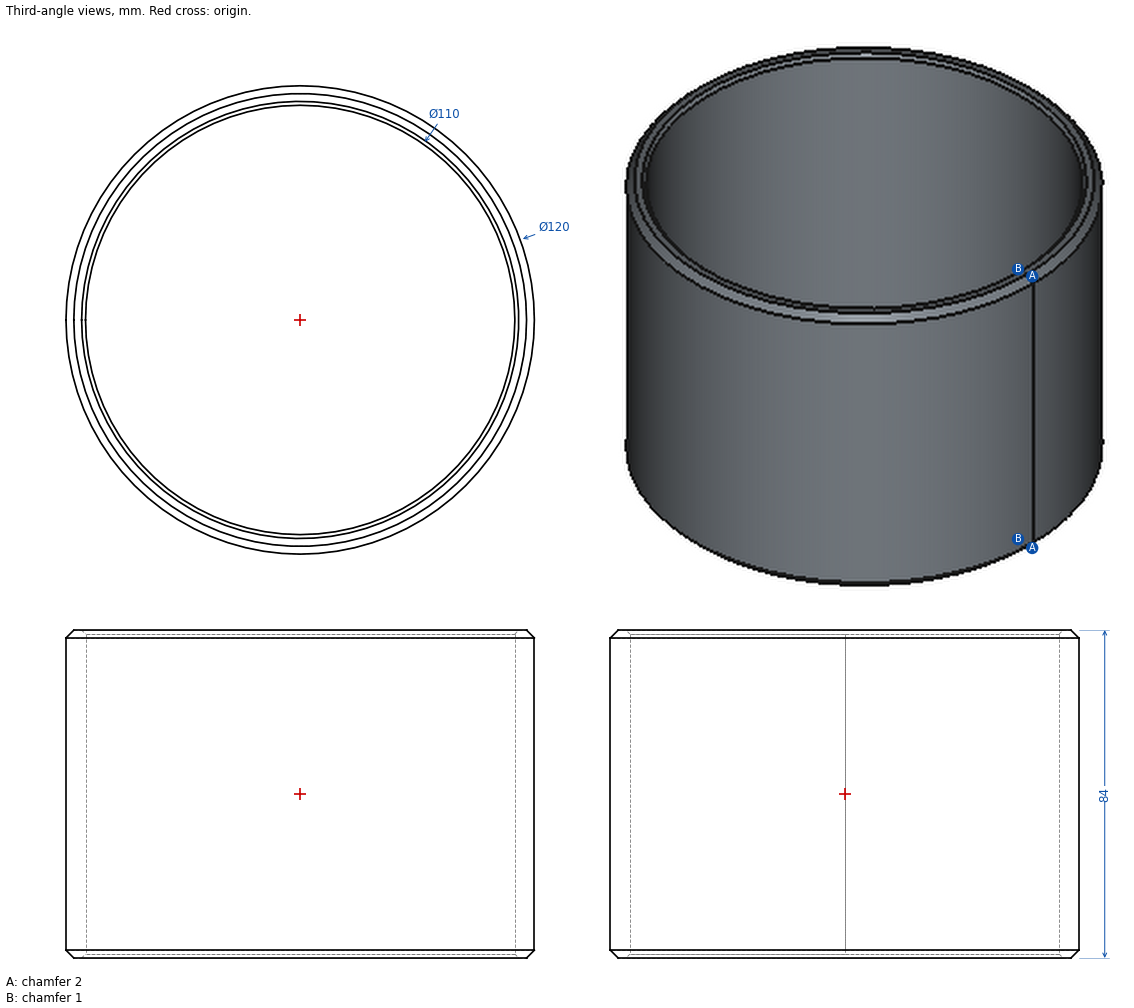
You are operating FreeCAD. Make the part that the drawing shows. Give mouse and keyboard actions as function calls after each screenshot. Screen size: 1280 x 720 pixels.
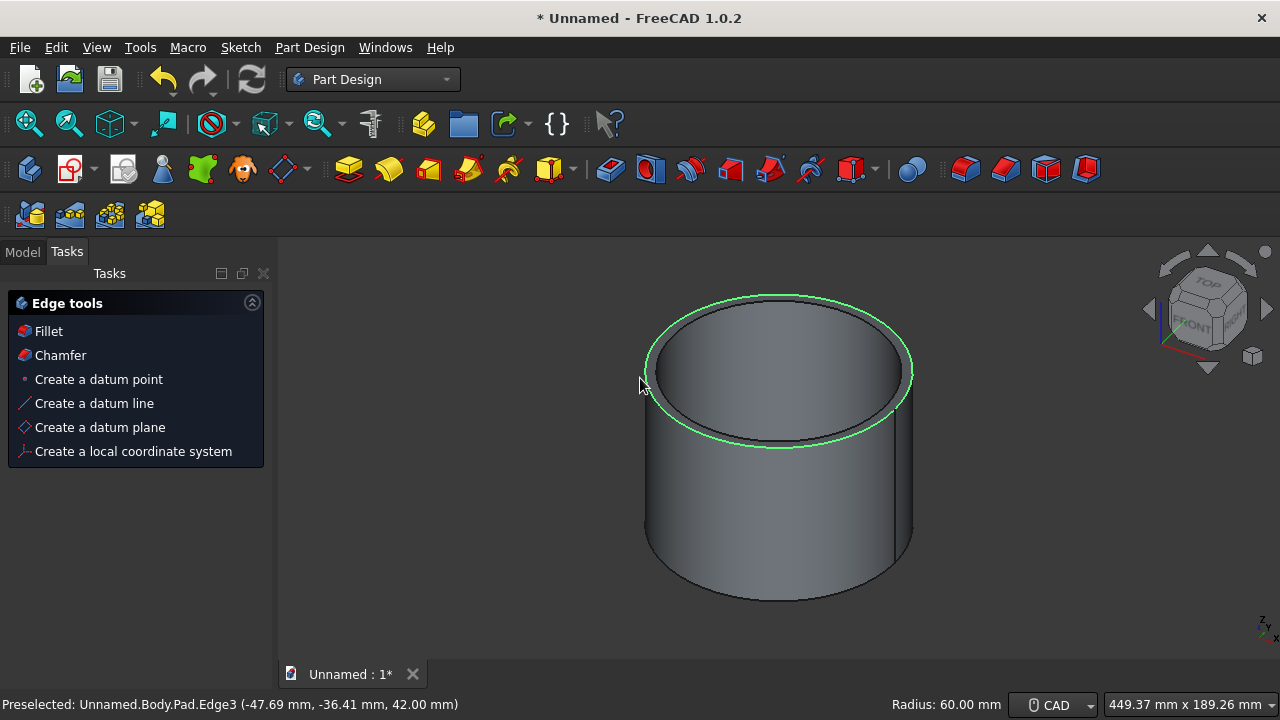
key(0)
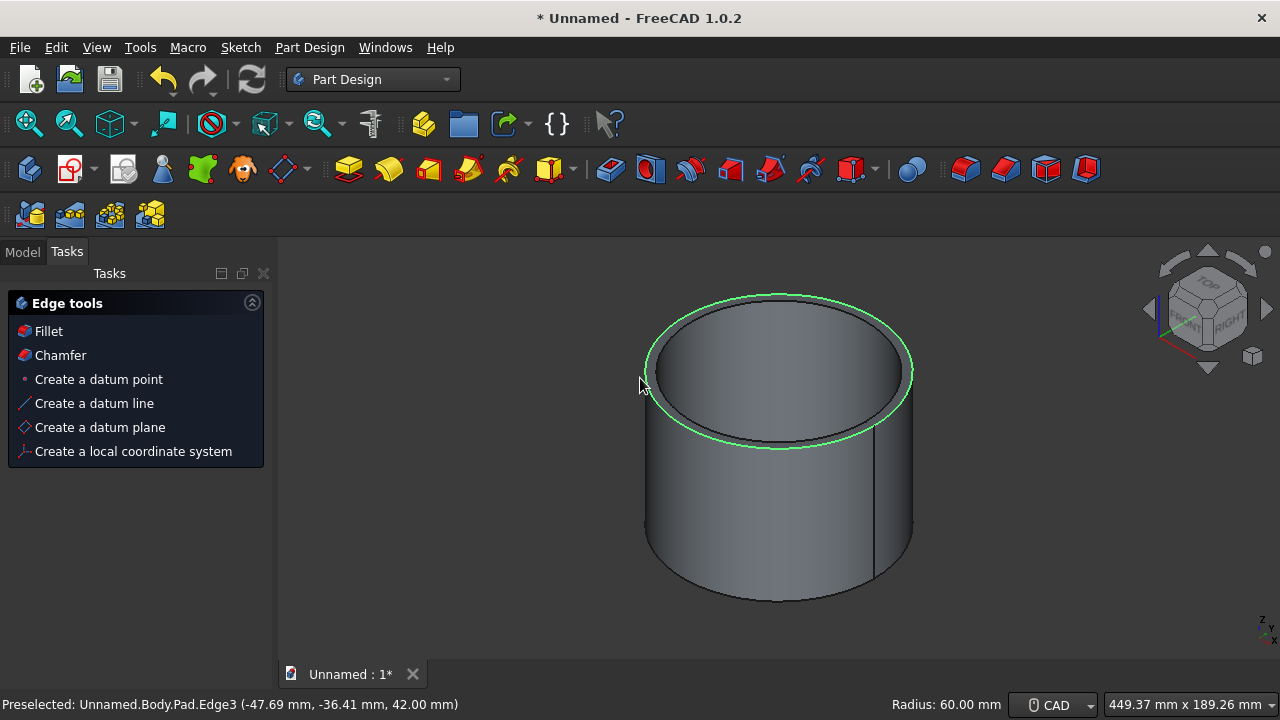
key(2)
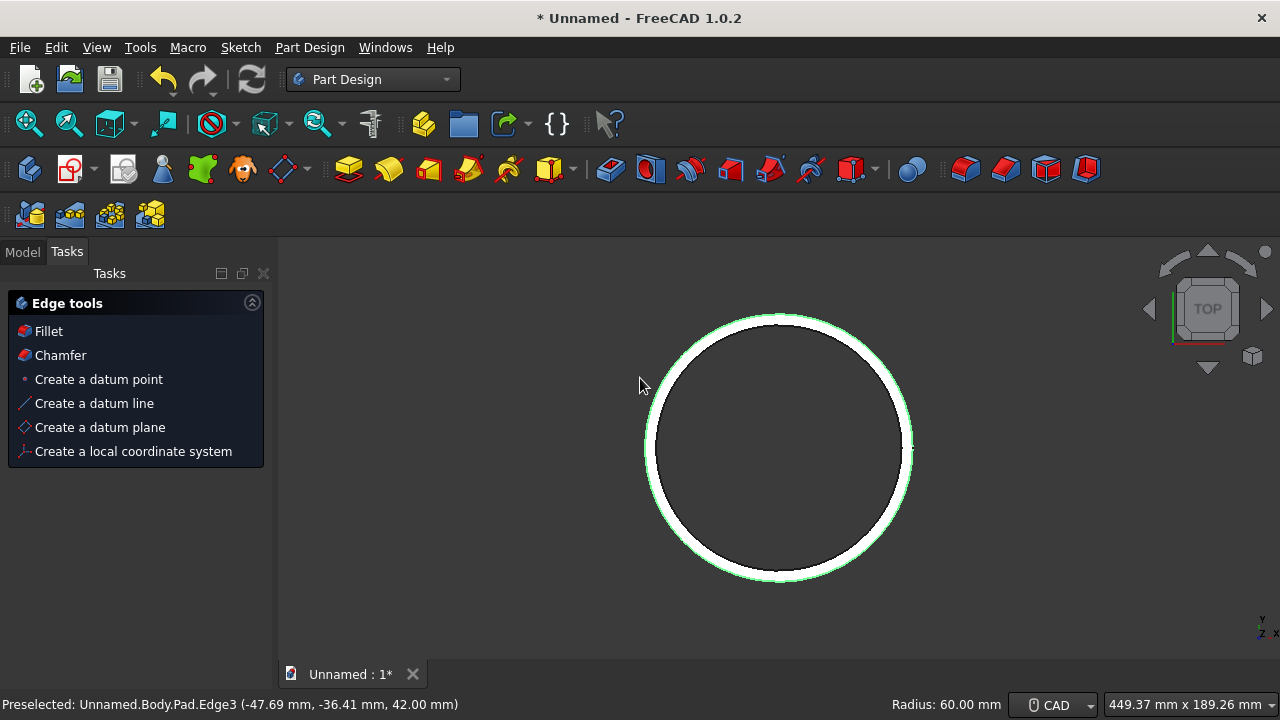
key(1)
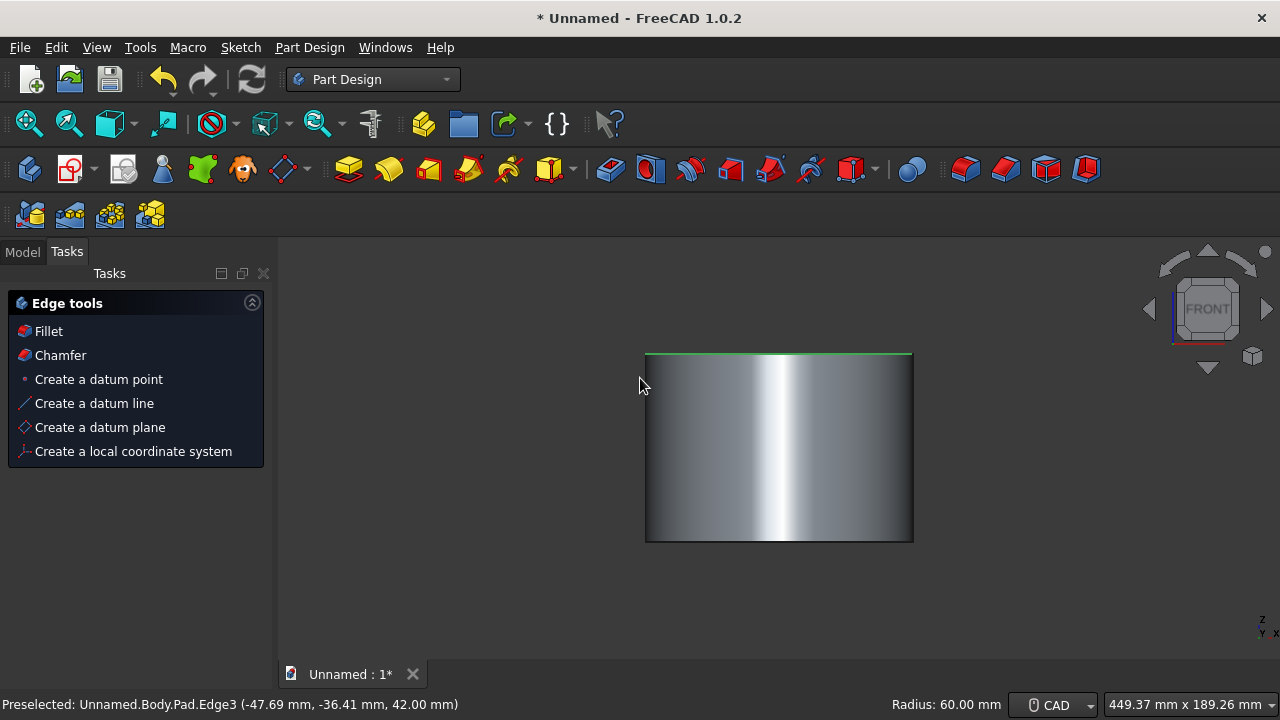
key(v)
key(f)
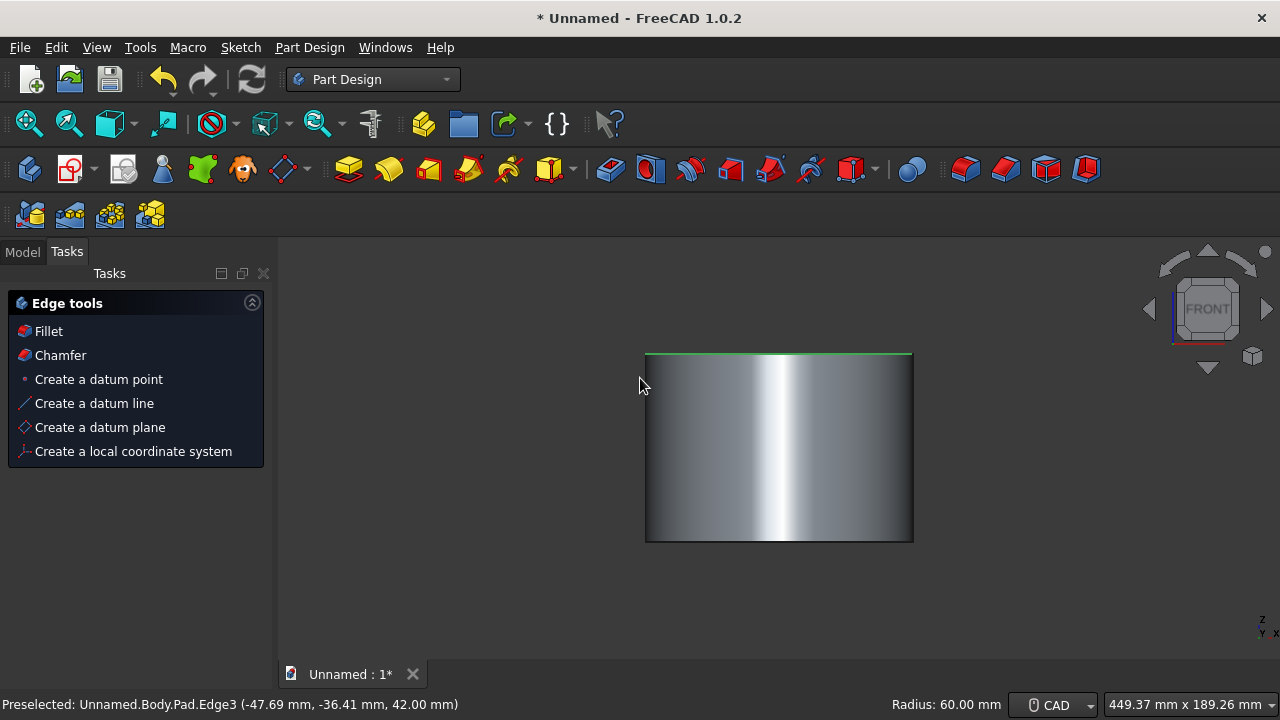
click(671, 541, ctrl)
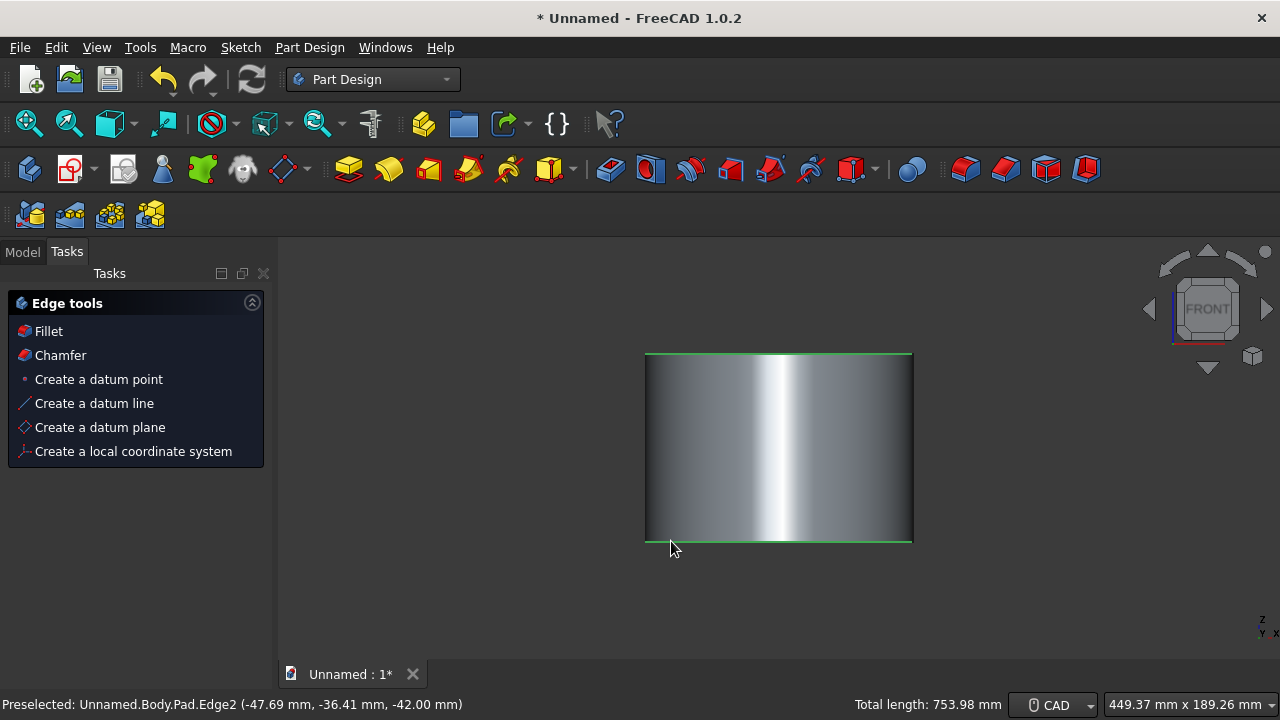
click(1006, 170)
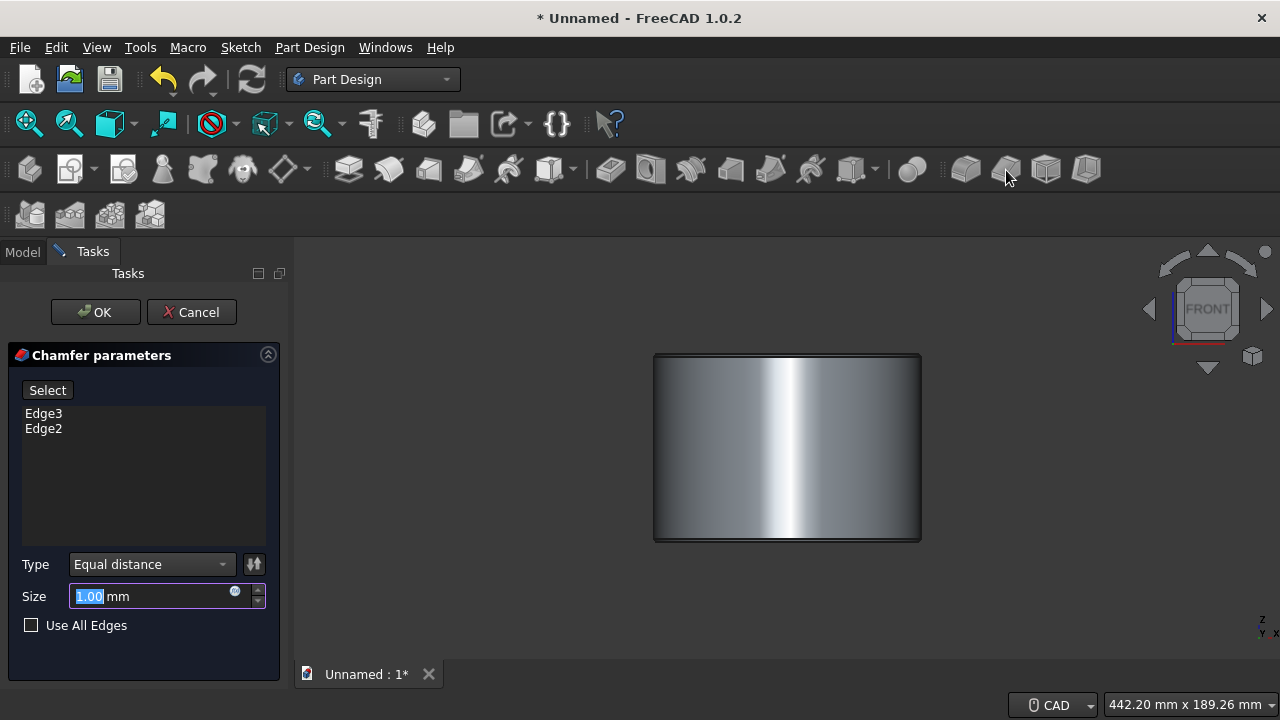
text(2)
key(Tab)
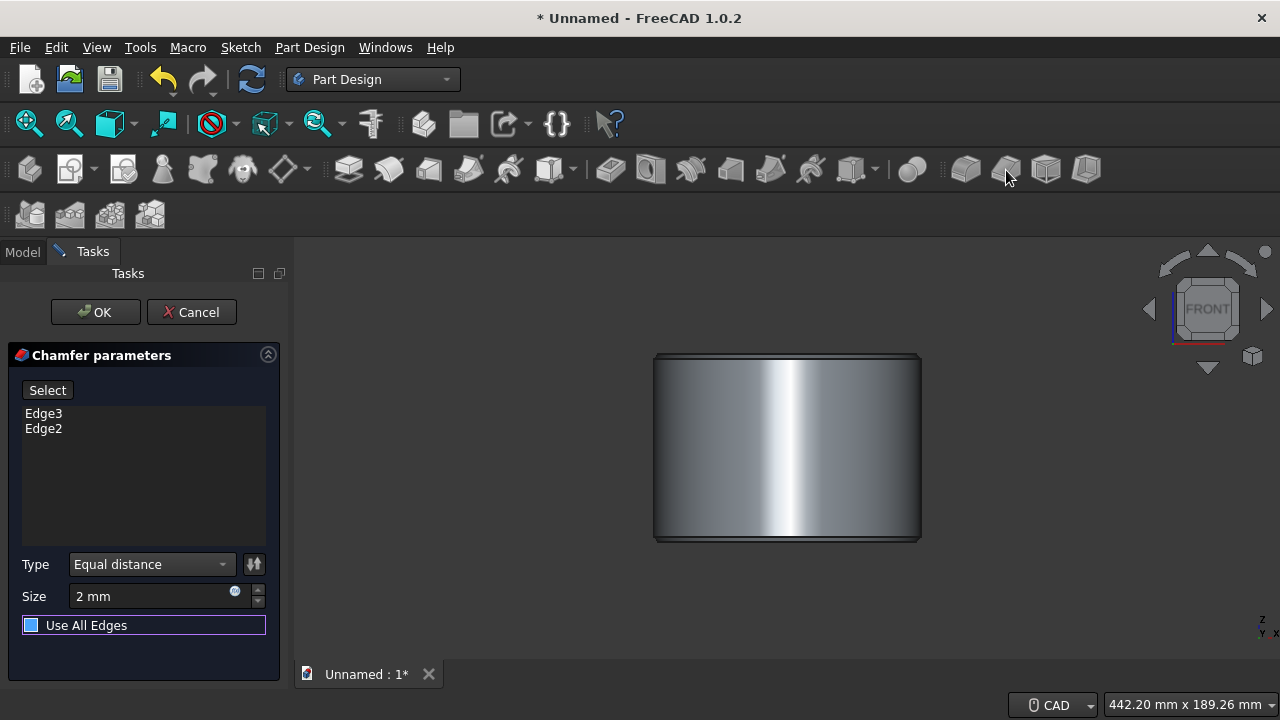
click(96, 312)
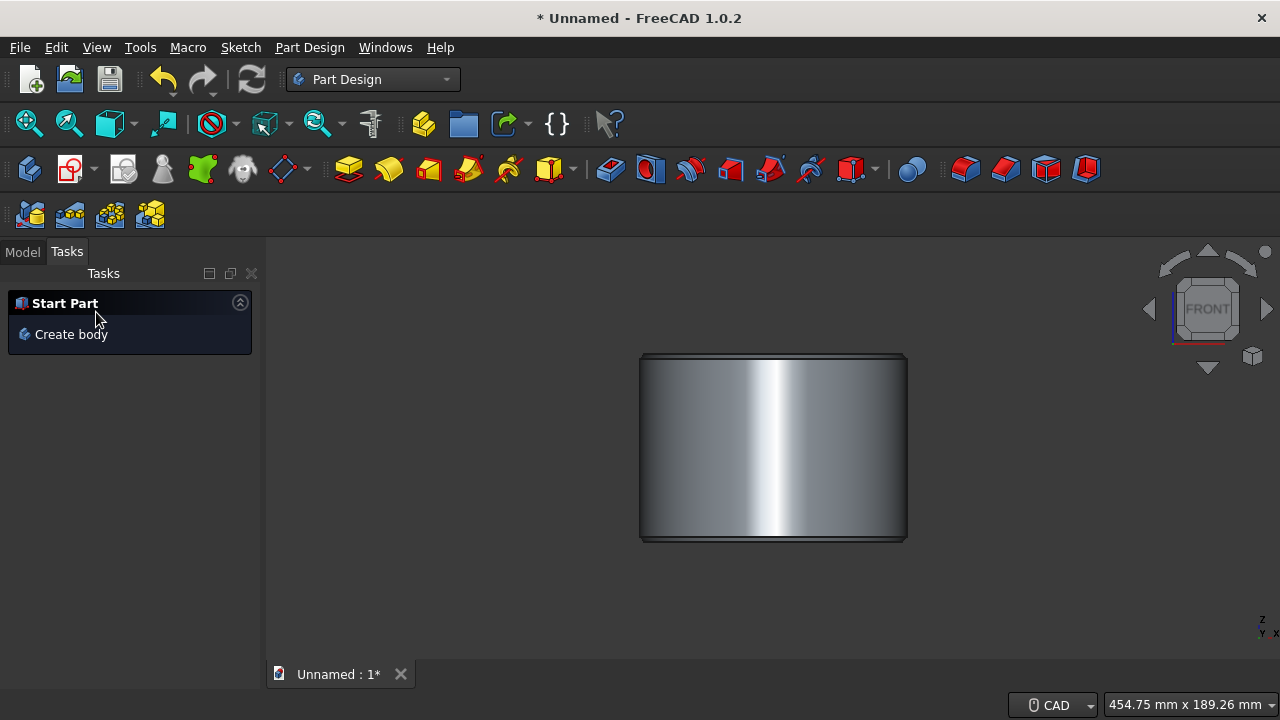
click(30, 124)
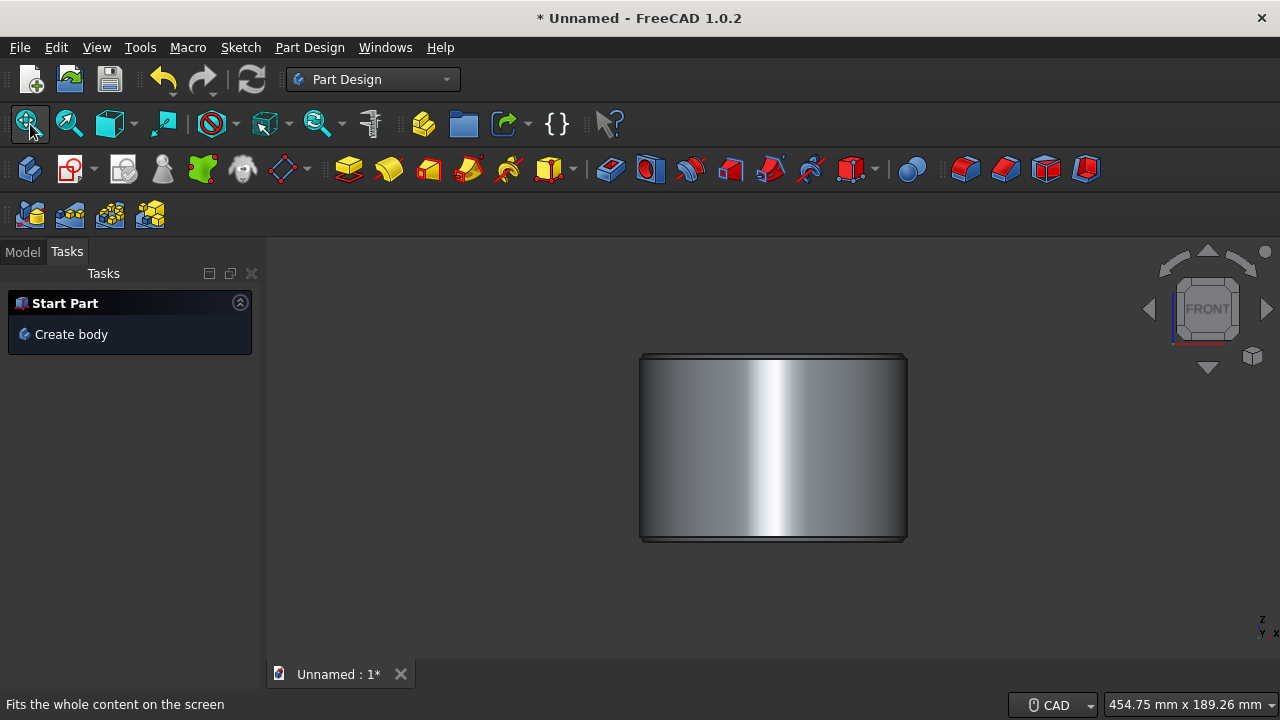
key(0)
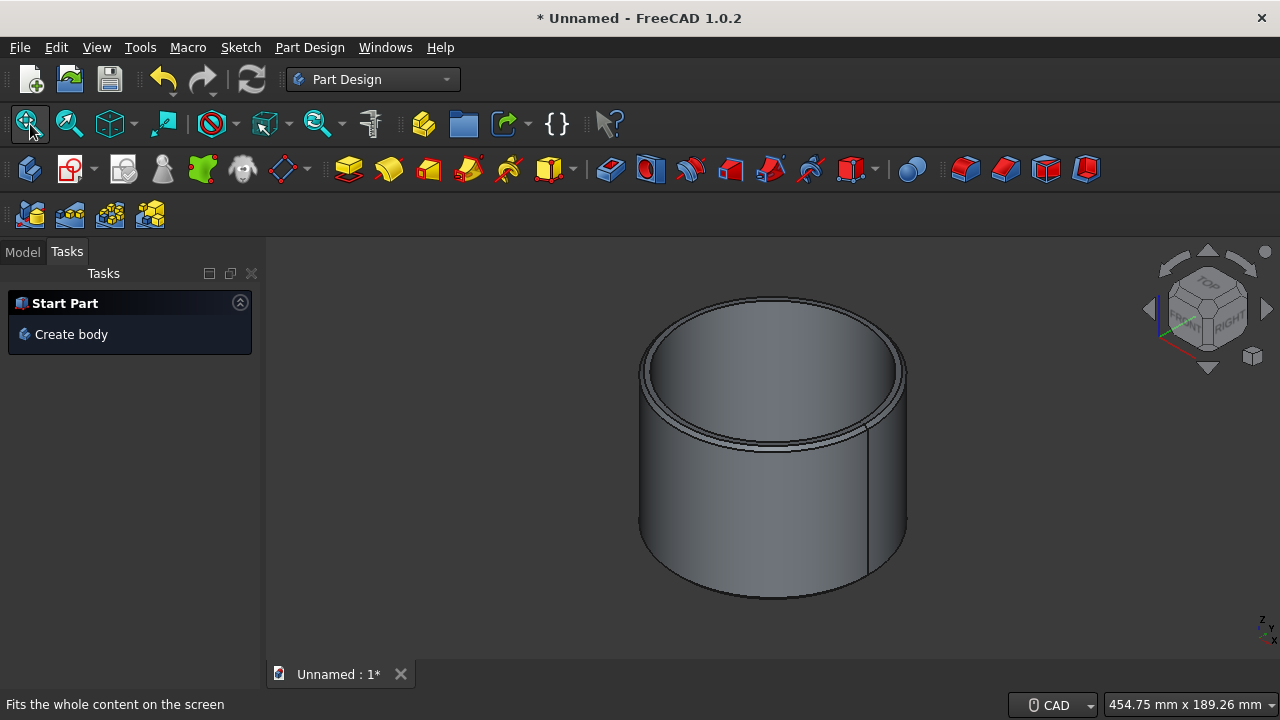
click(686, 320)